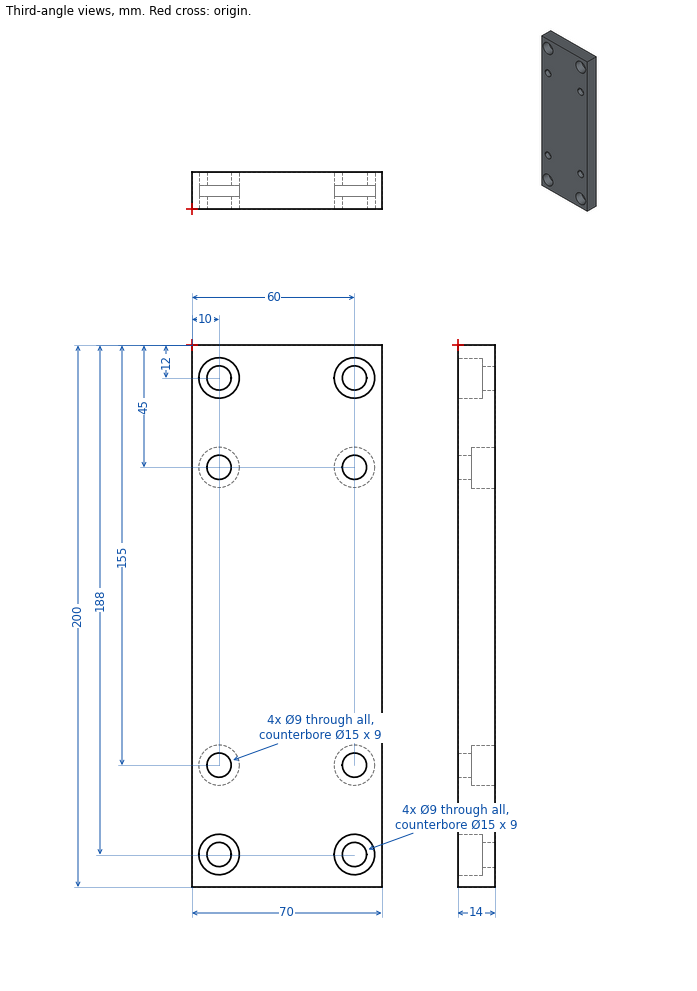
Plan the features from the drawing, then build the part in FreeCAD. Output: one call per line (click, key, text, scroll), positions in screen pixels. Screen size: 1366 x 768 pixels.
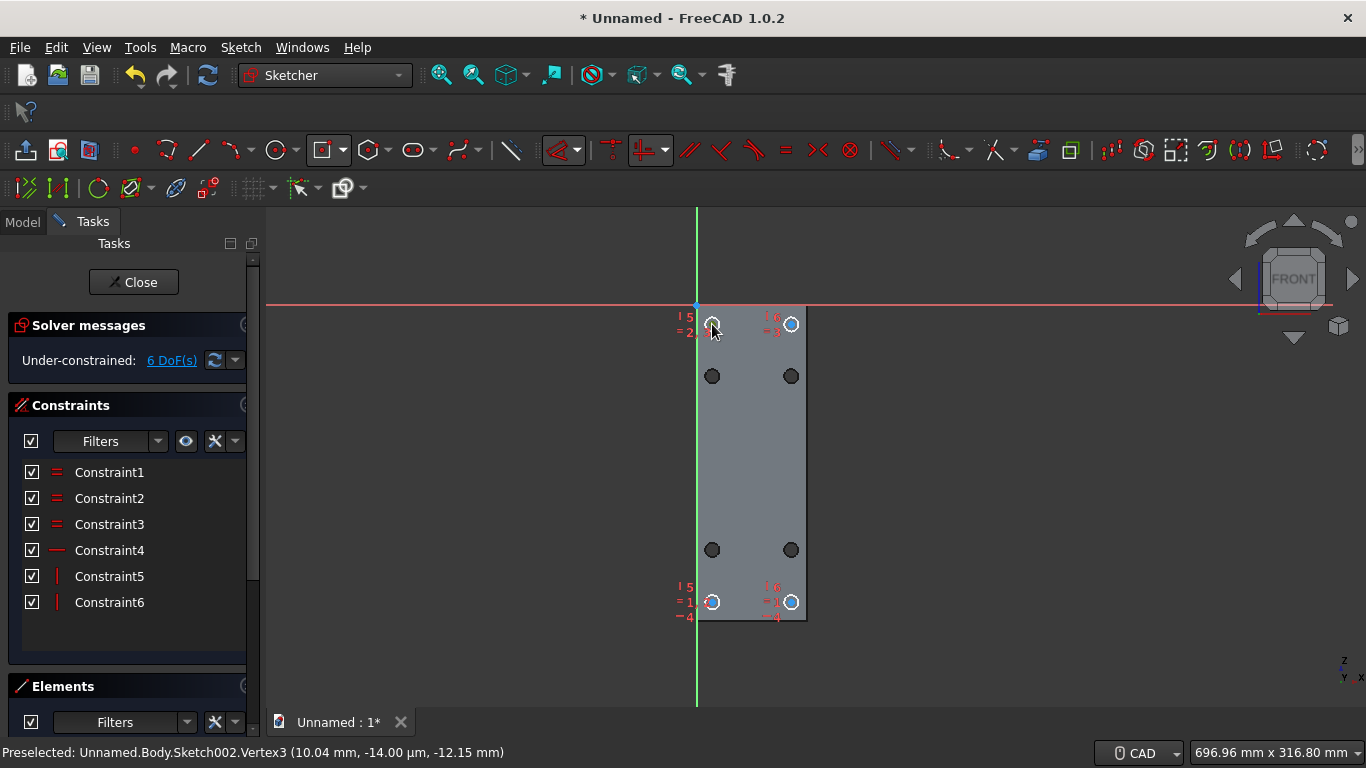
click(791, 324)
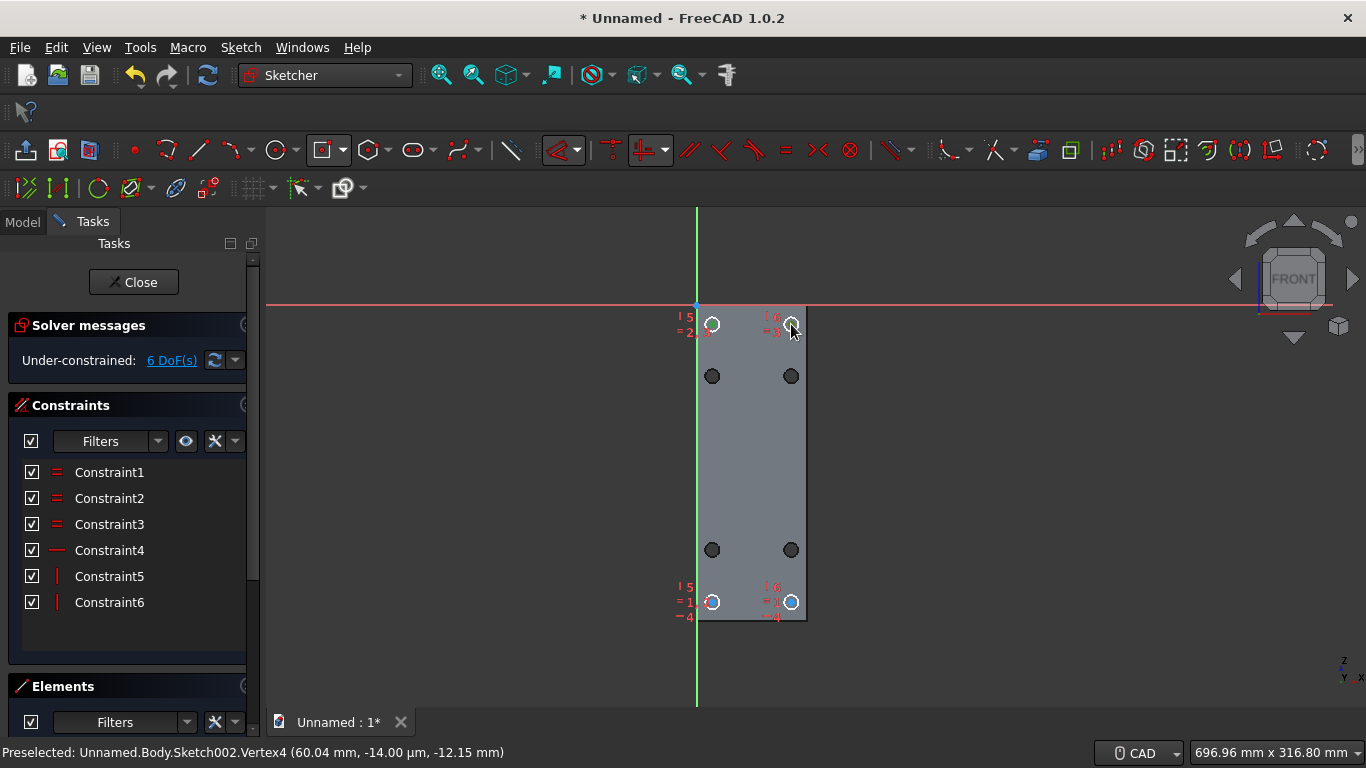
key(h)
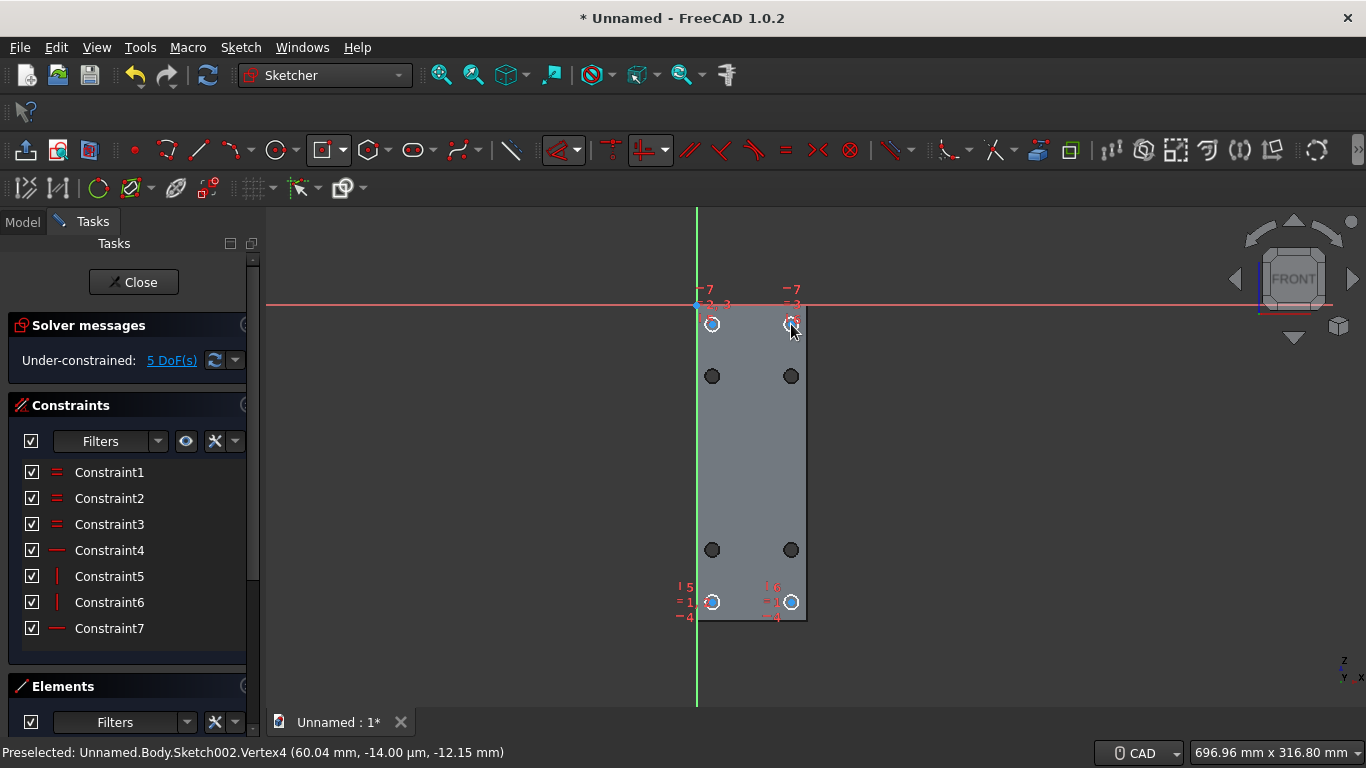
key(d)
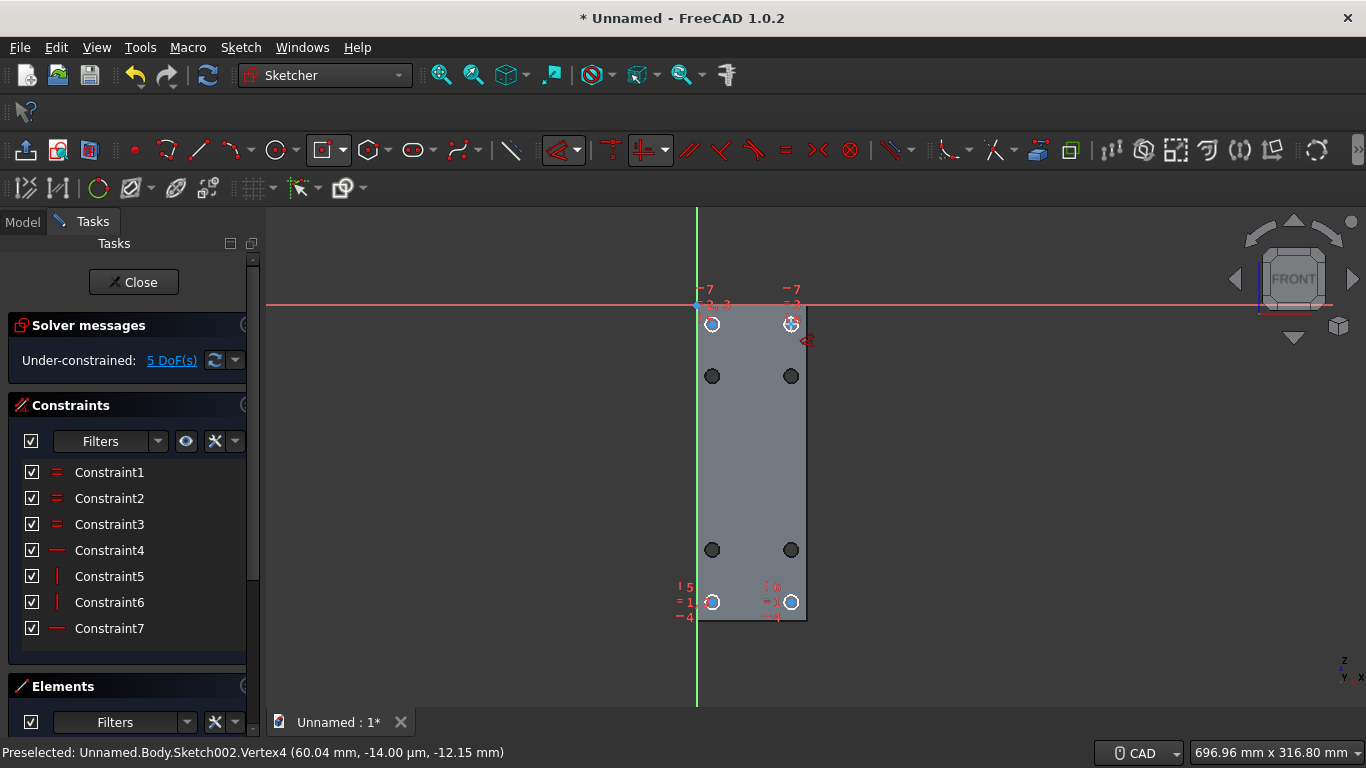
scroll(796, 597, up, 6)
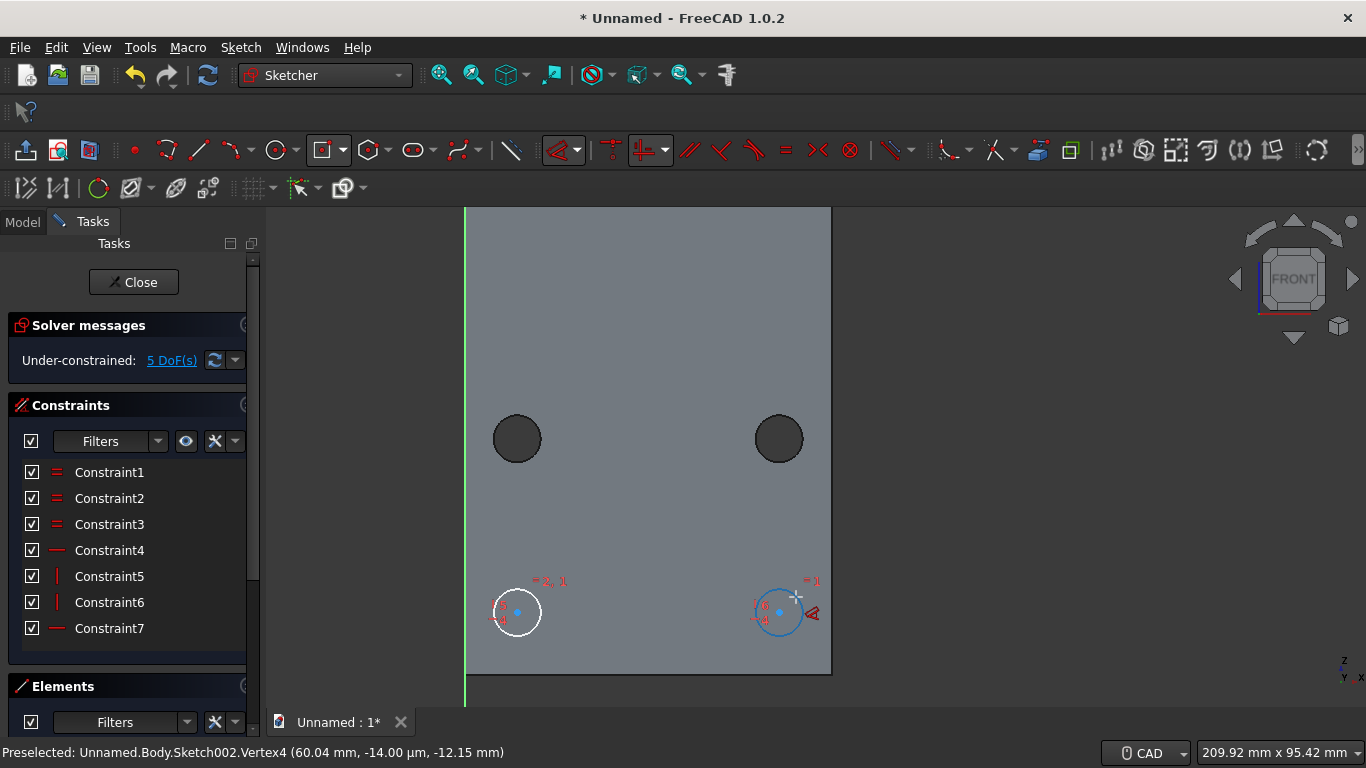
click(796, 596)
click(819, 573)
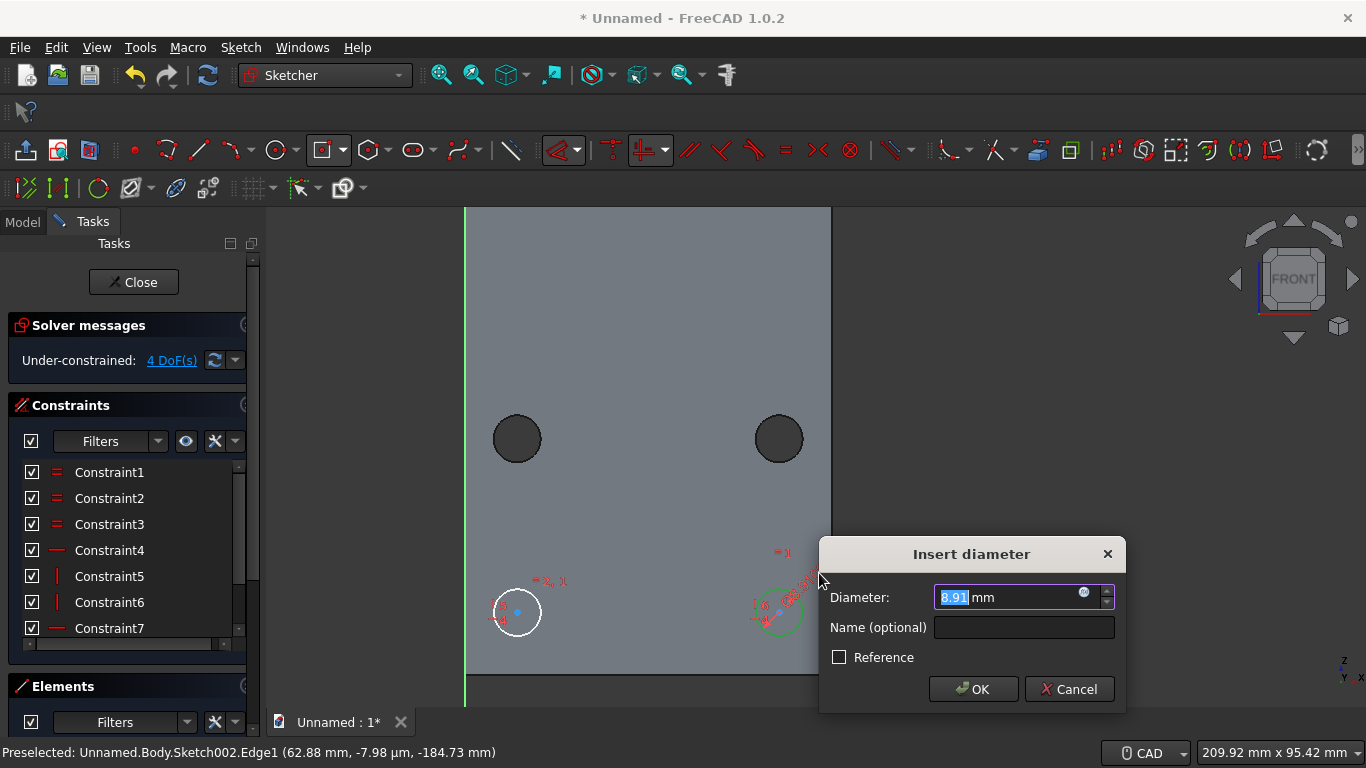
text(9)
key(Return)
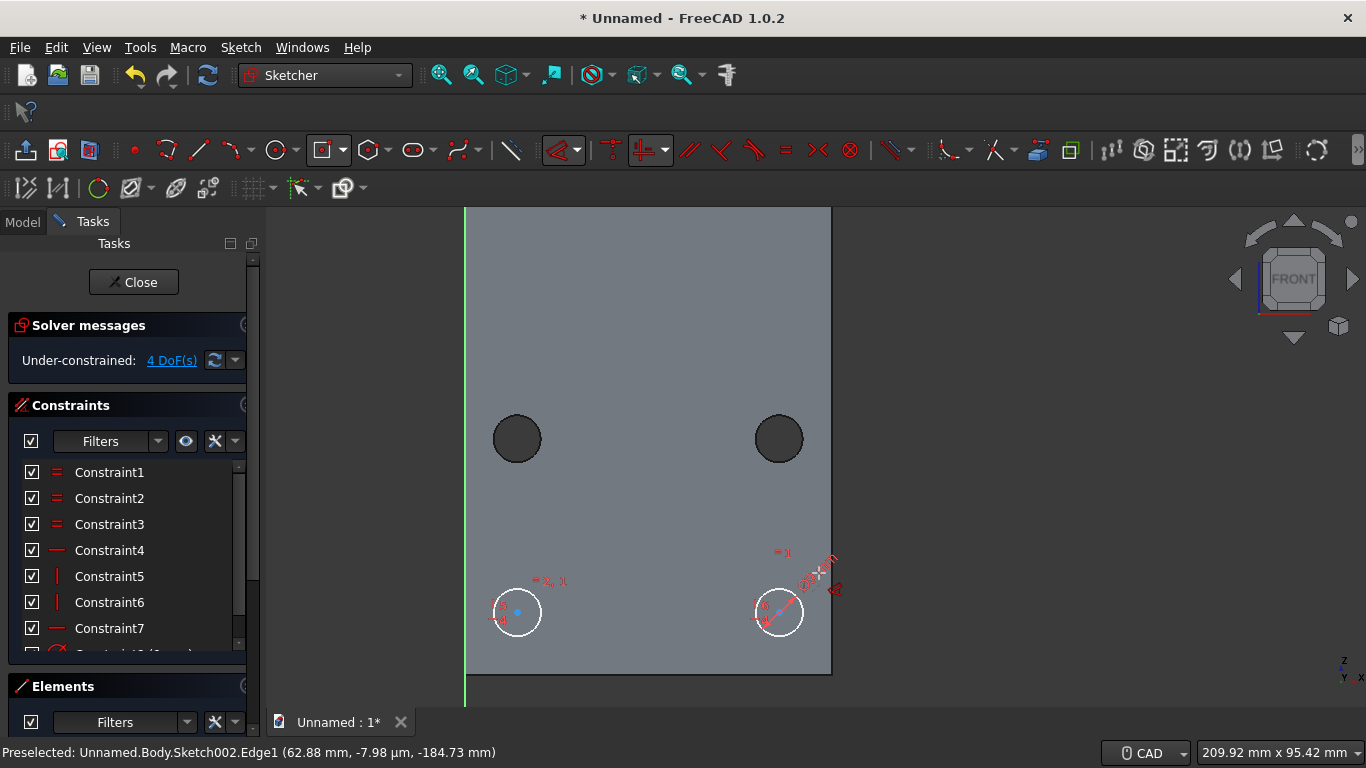
click(779, 613)
click(622, 647)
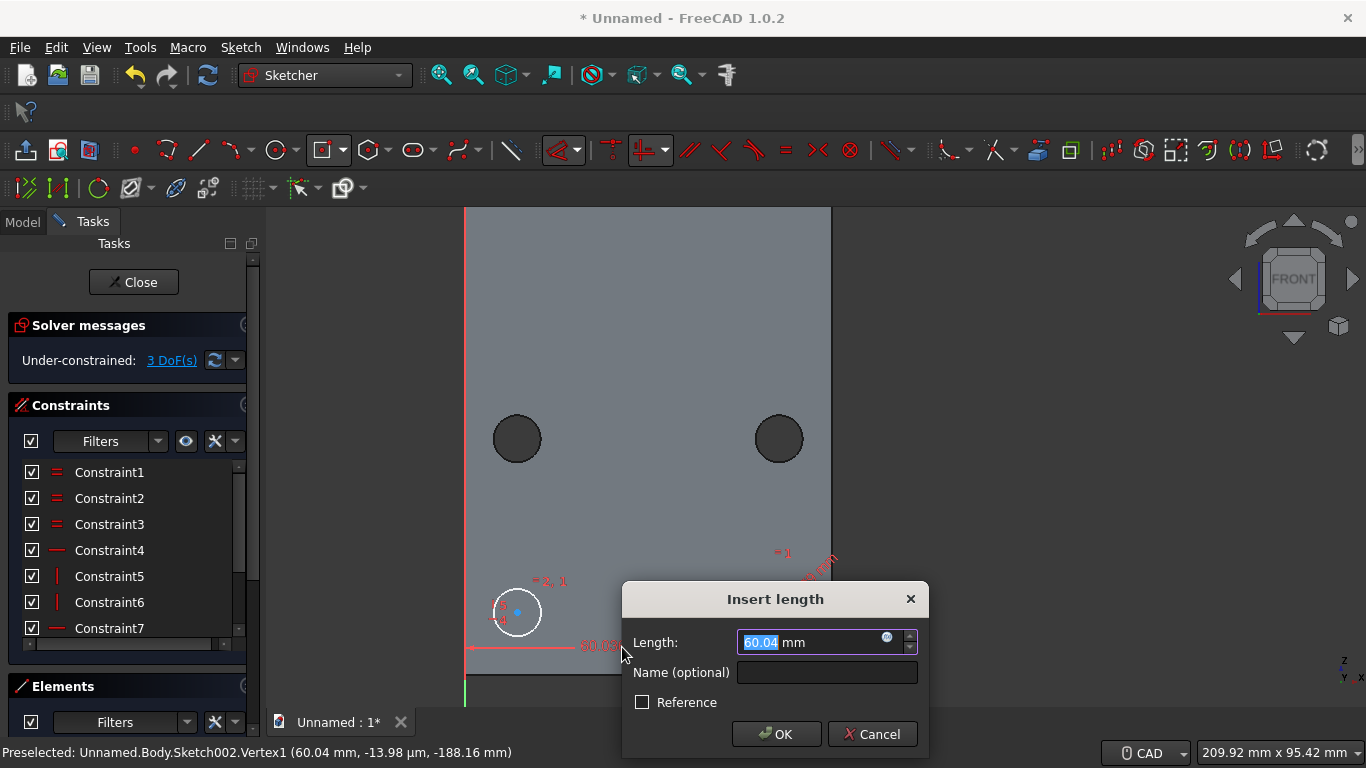
text(60)
key(Return)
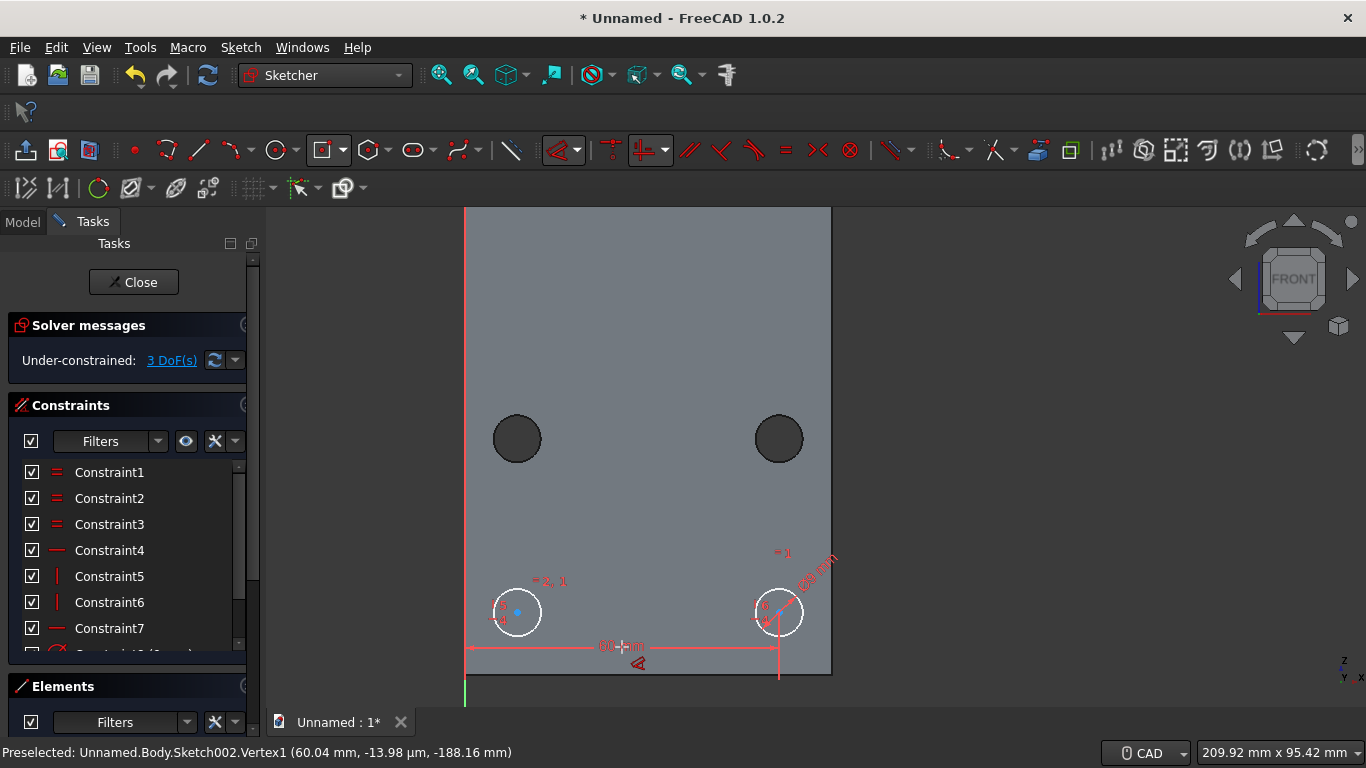
click(517, 613)
click(491, 647)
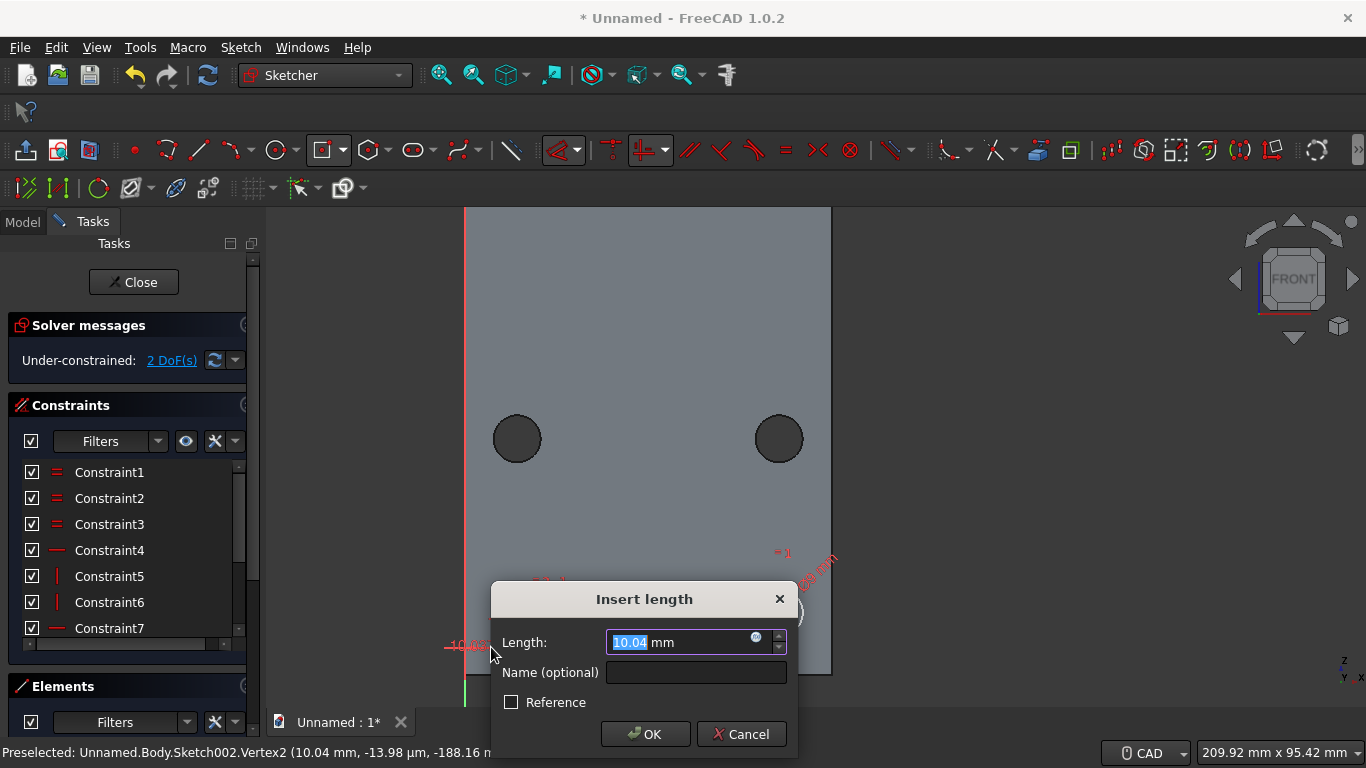
text(10)
key(Return)